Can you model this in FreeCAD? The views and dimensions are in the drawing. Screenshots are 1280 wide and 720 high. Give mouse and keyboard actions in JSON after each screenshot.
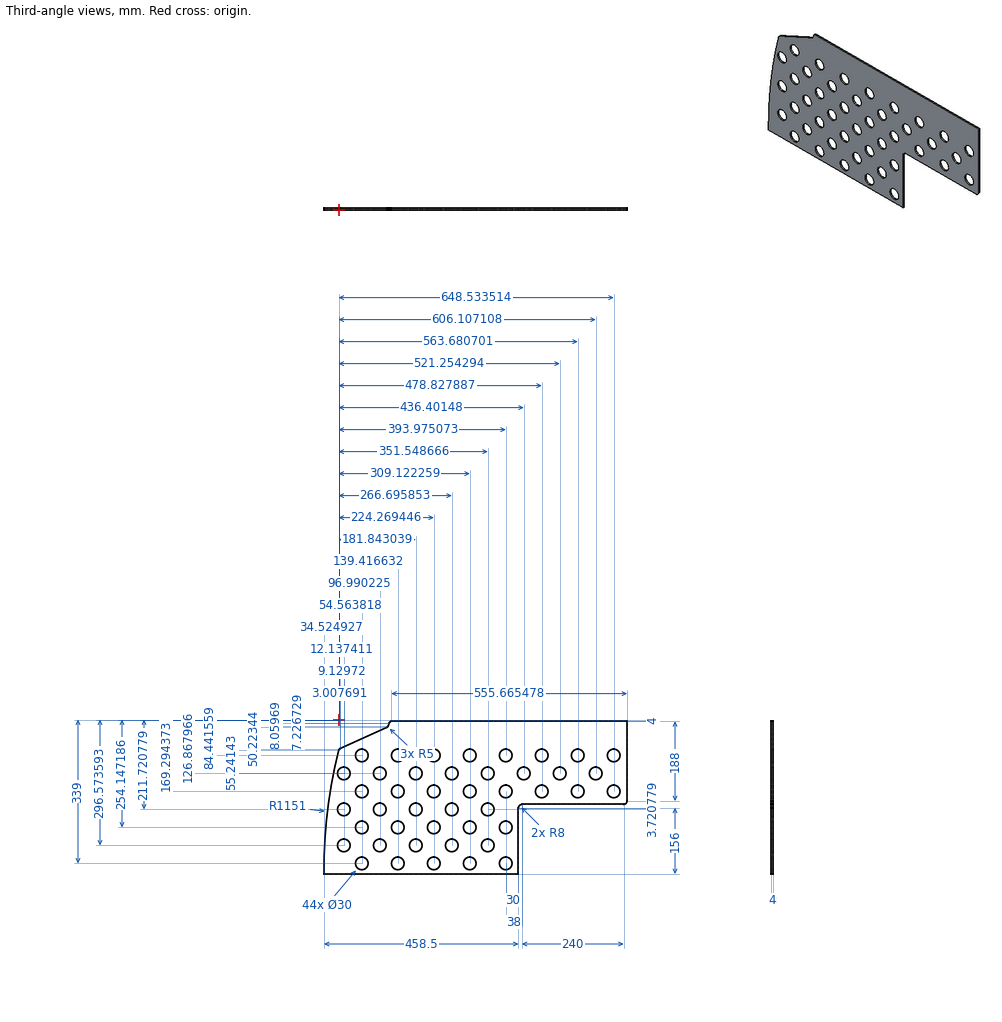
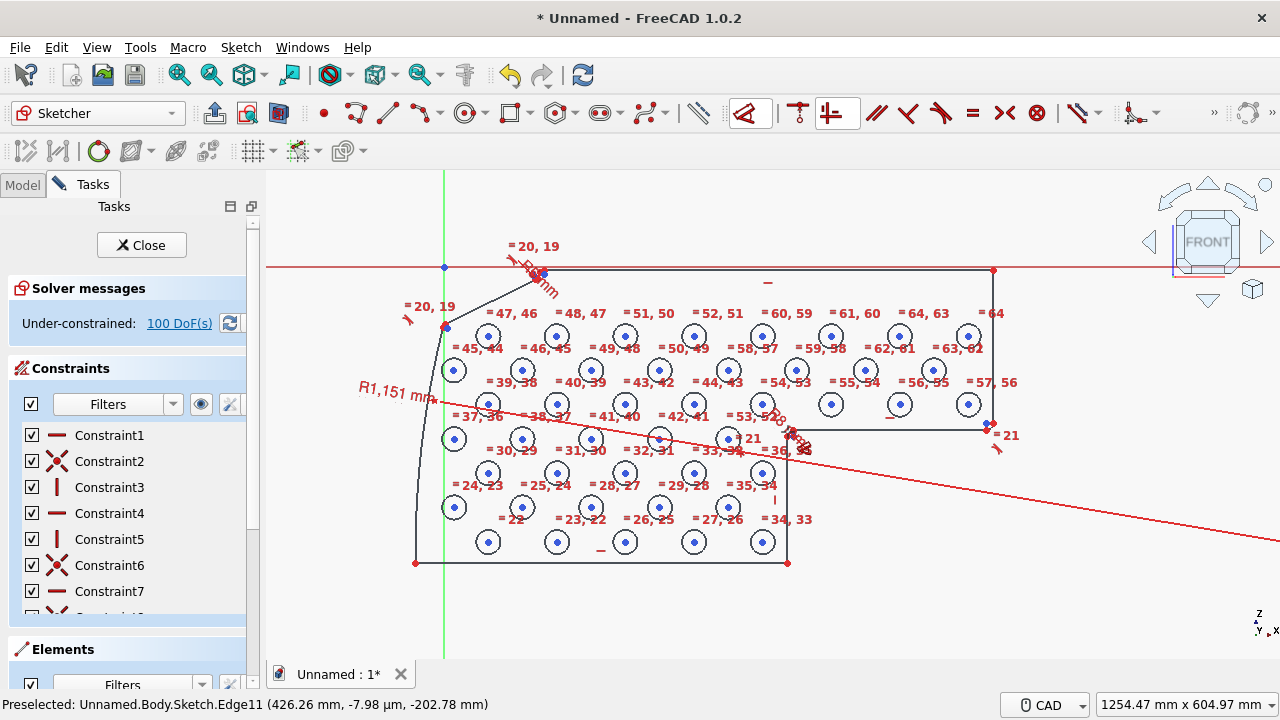
{"action": "scroll", "coordinate": [497, 534], "scroll_direction": "up", "scroll_amount": 3}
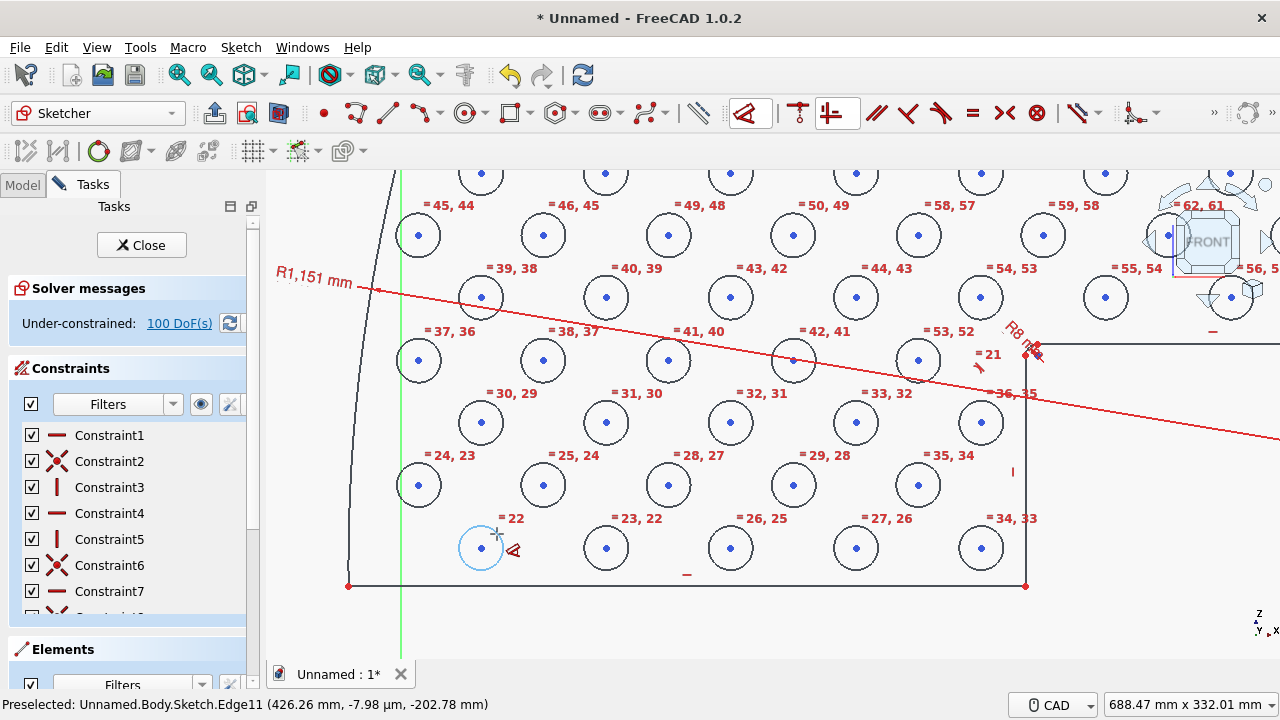
{"action": "left_click", "coordinate": [497, 532]}
{"action": "left_click", "coordinate": [533, 532]}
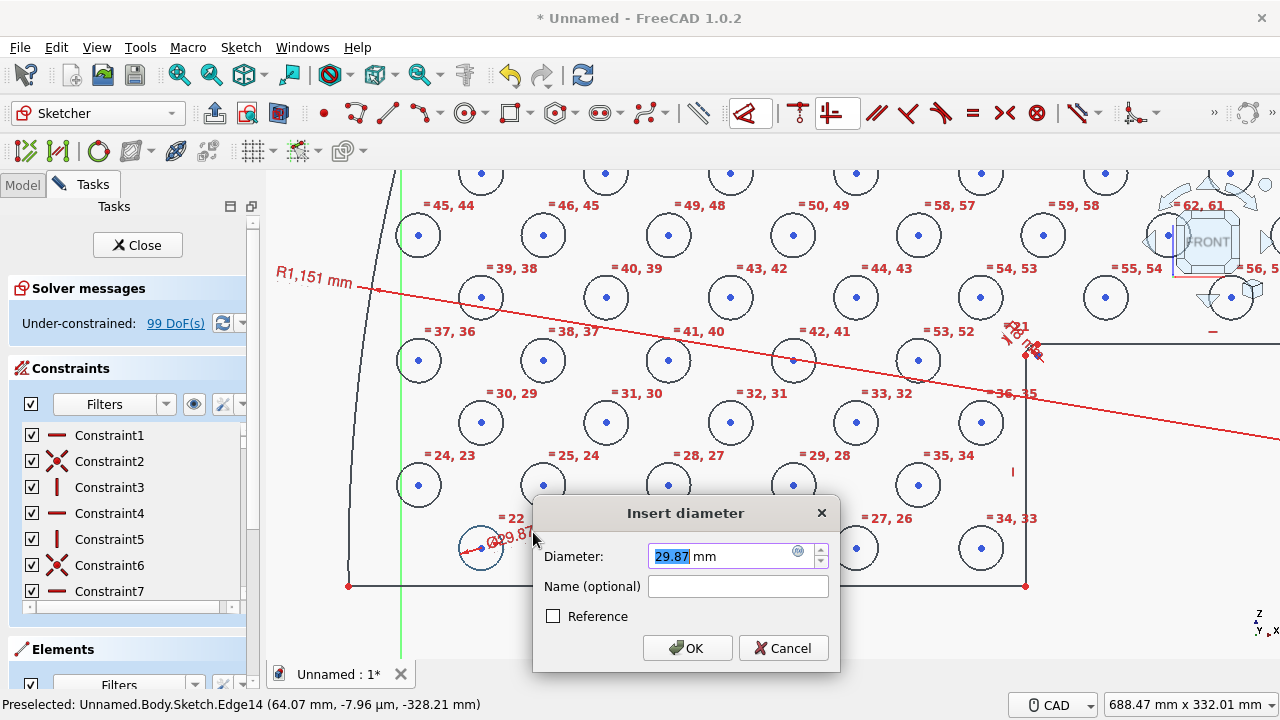
{"action": "type", "text": "30"}
{"action": "key", "text": "Return"}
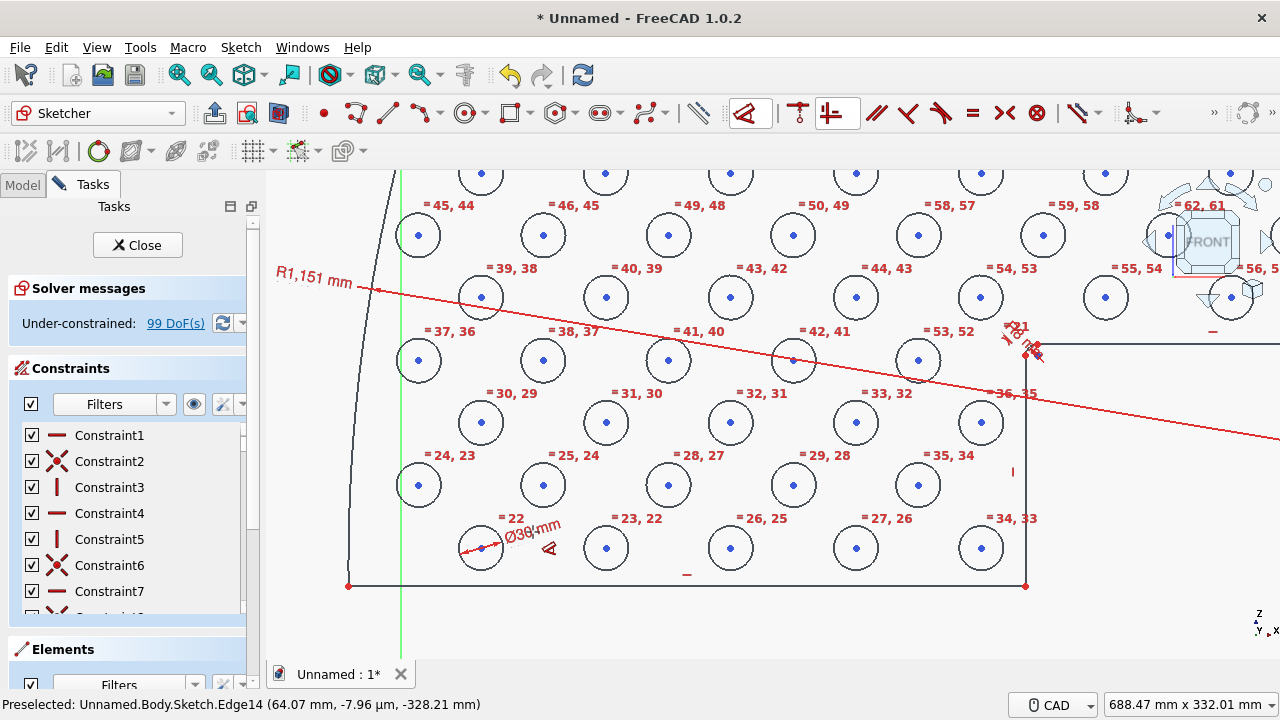
{"action": "scroll", "coordinate": [496, 535], "scroll_direction": "down", "scroll_amount": 3}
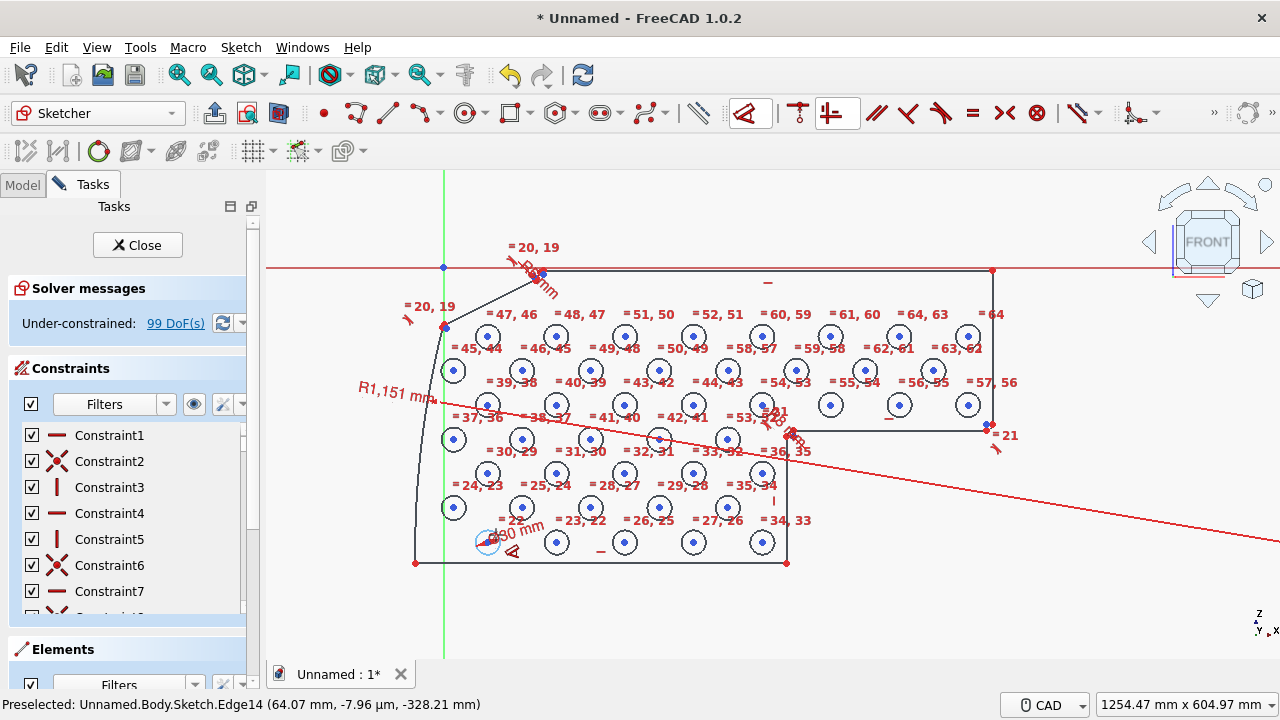
{"action": "scroll", "coordinate": [993, 271], "scroll_direction": "up", "scroll_amount": 13}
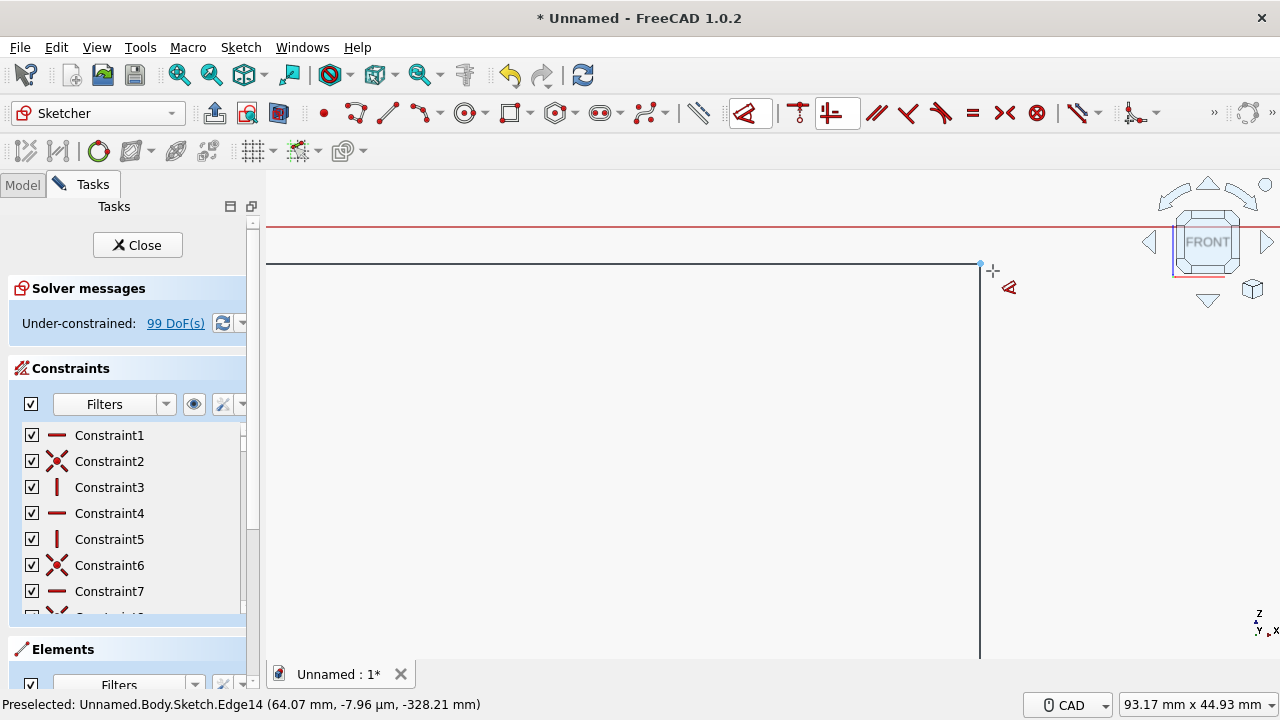
{"action": "left_click", "coordinate": [980, 264]}
{"action": "left_click", "coordinate": [1014, 245]}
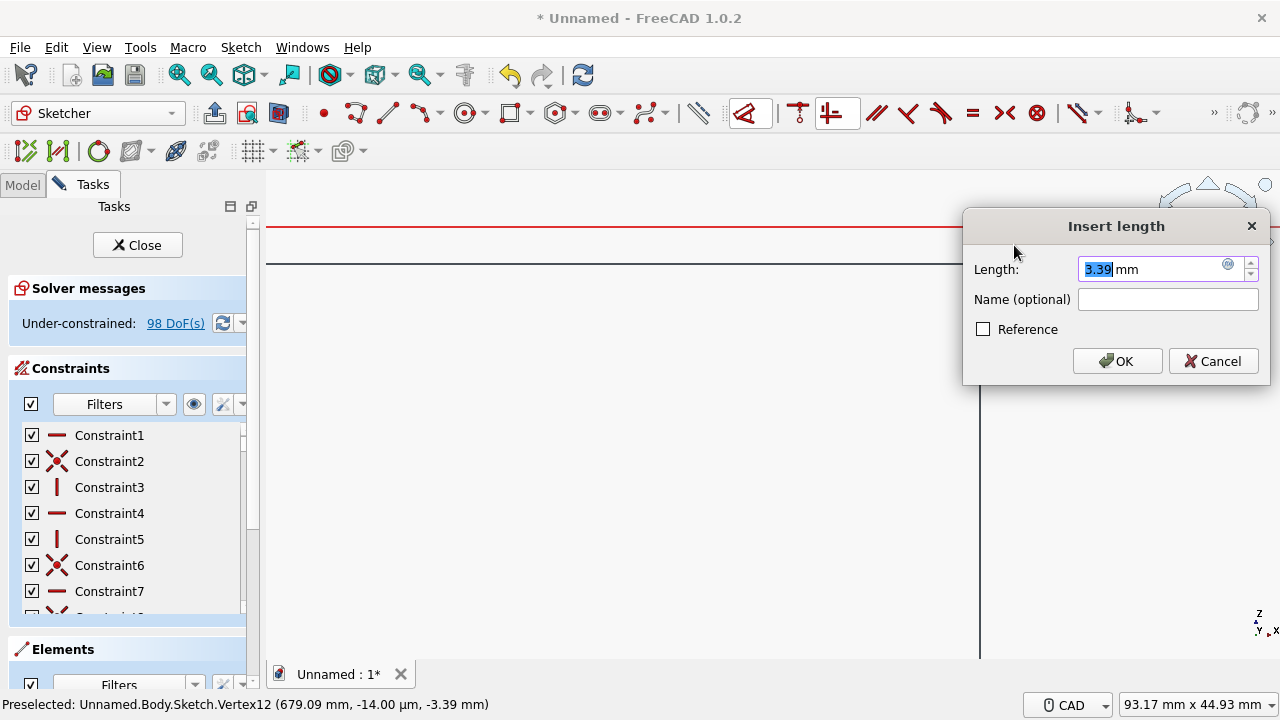
{"action": "type", "text": "4"}
{"action": "key", "text": "Return"}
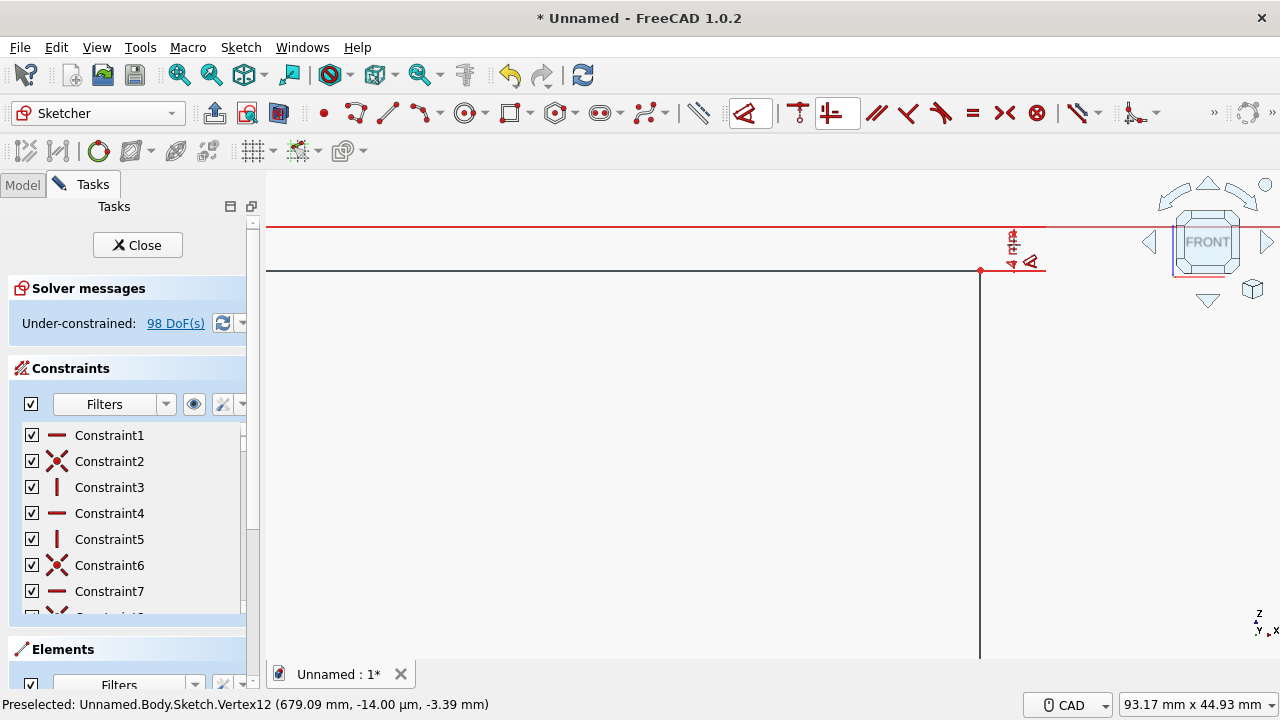
{"action": "scroll", "coordinate": [994, 271], "scroll_direction": "down", "scroll_amount": 13}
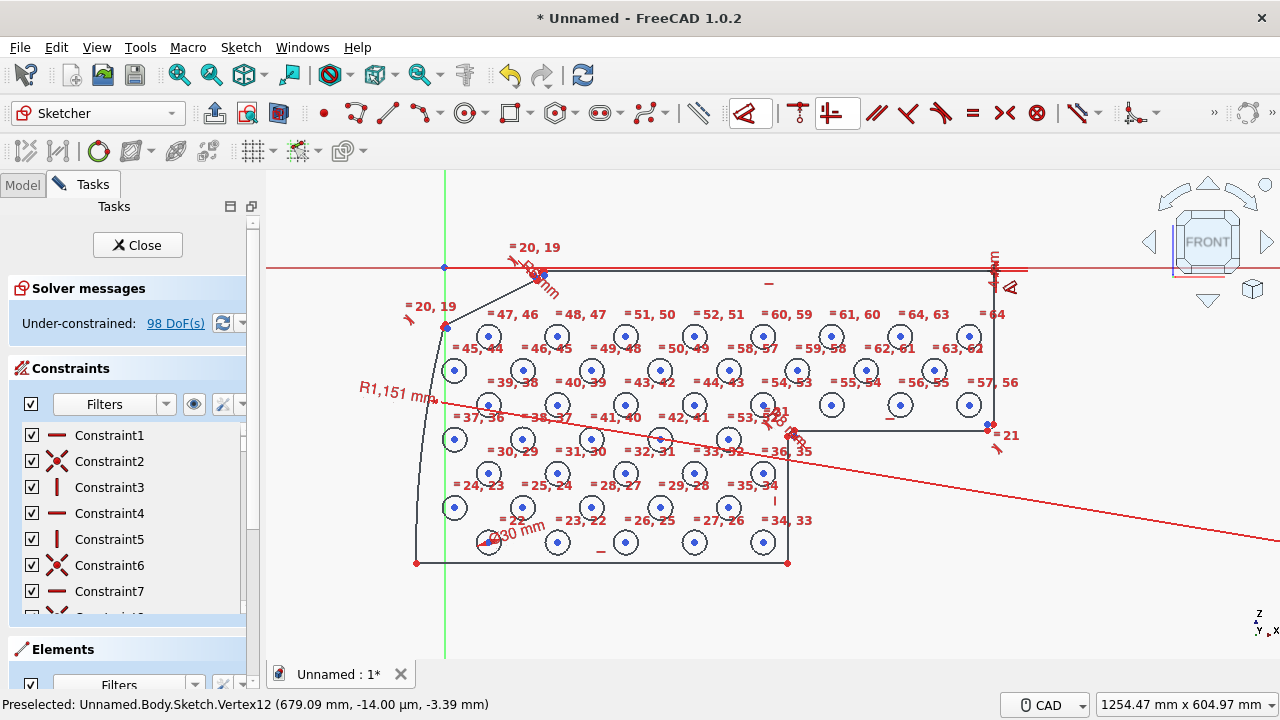
{"action": "left_click", "coordinate": [788, 526]}
{"action": "left_click", "coordinate": [822, 500]}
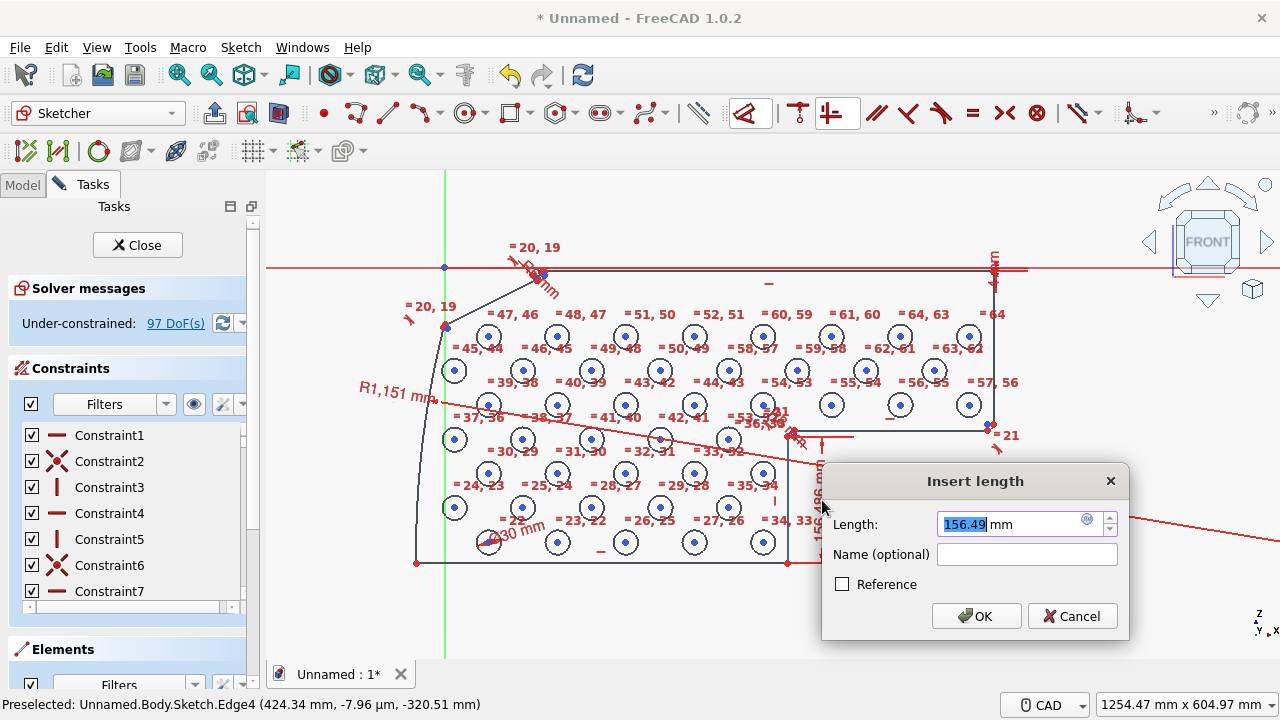
{"action": "type", "text": "156"}
{"action": "key", "text": "Return"}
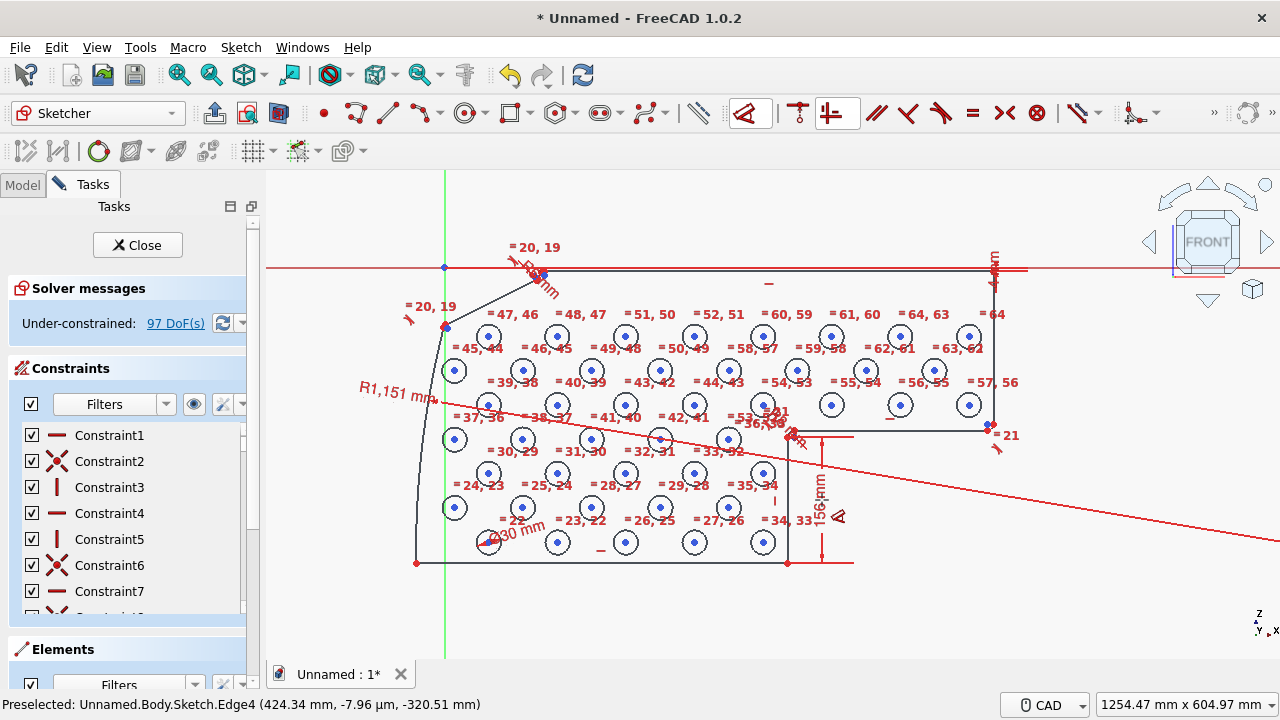
{"action": "left_click", "coordinate": [852, 431]}
{"action": "left_click", "coordinate": [891, 465]}